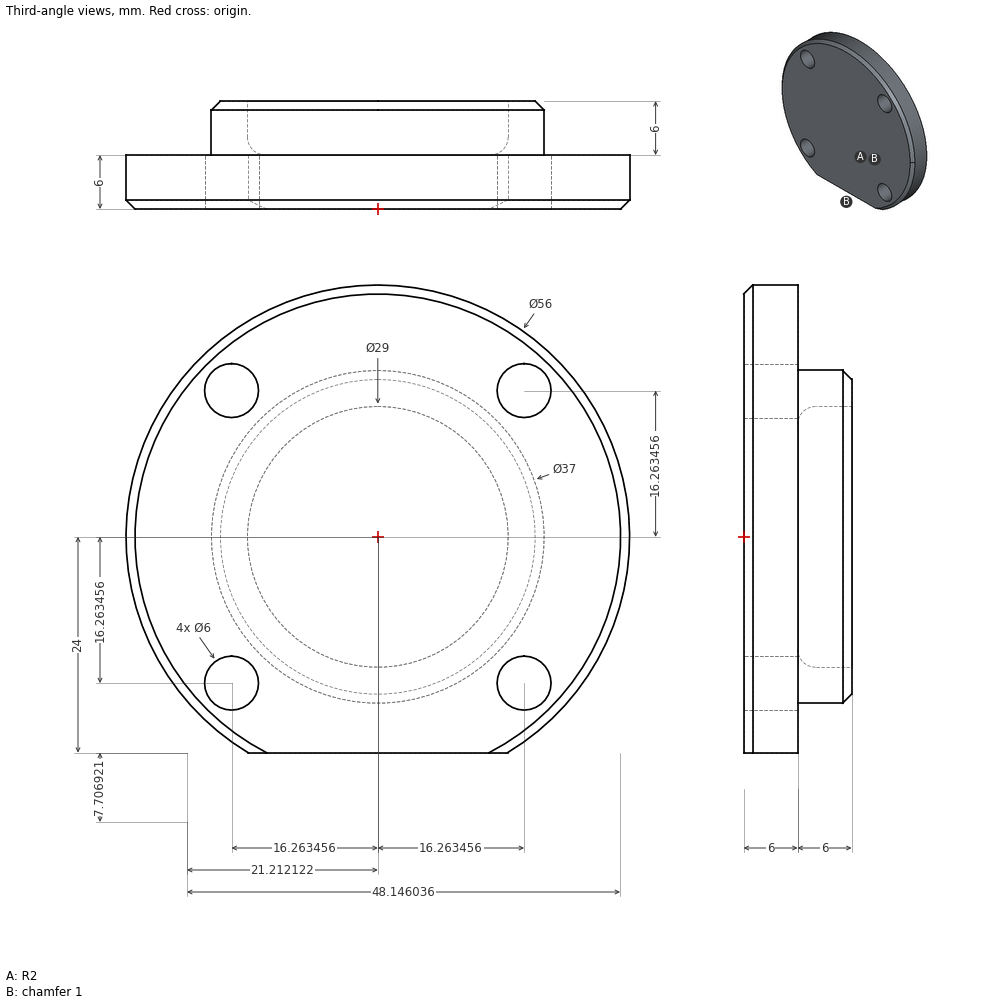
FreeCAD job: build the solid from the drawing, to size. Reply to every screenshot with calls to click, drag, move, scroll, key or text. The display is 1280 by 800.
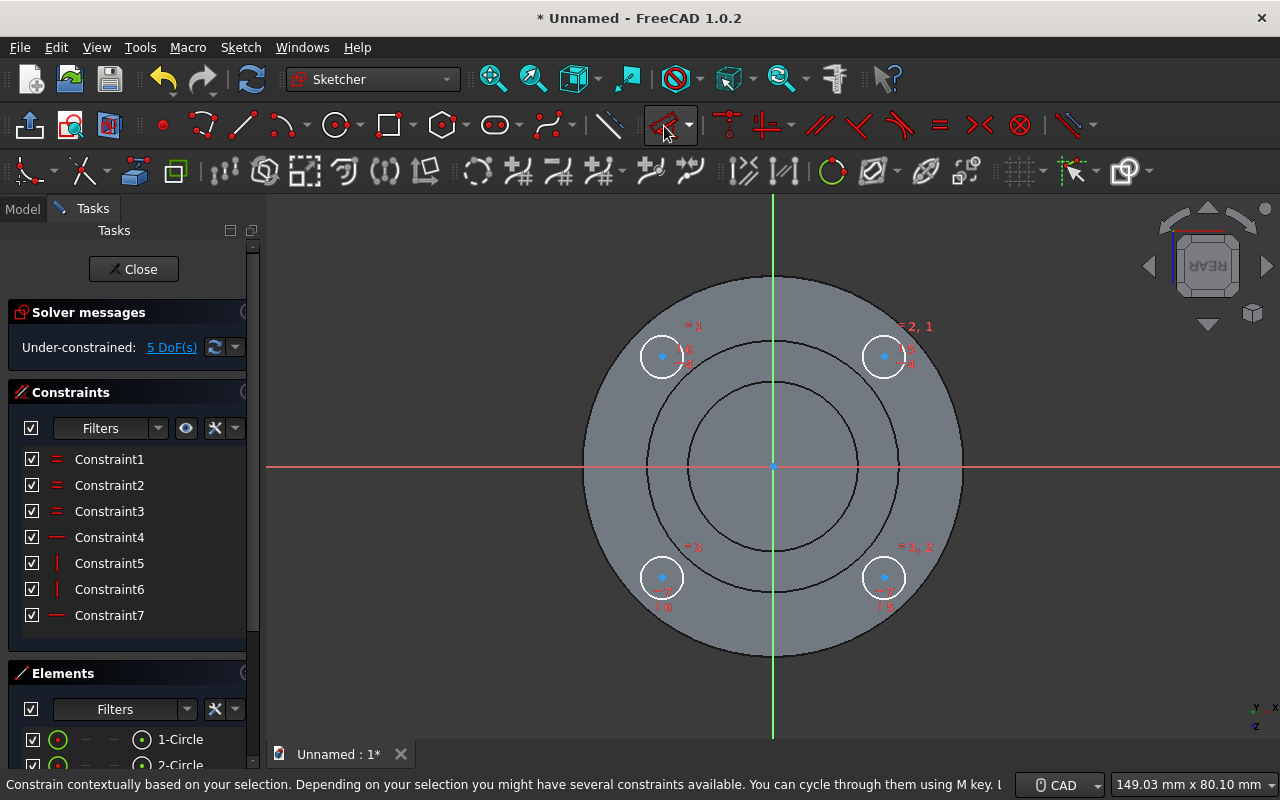
click(677, 342)
click(700, 319)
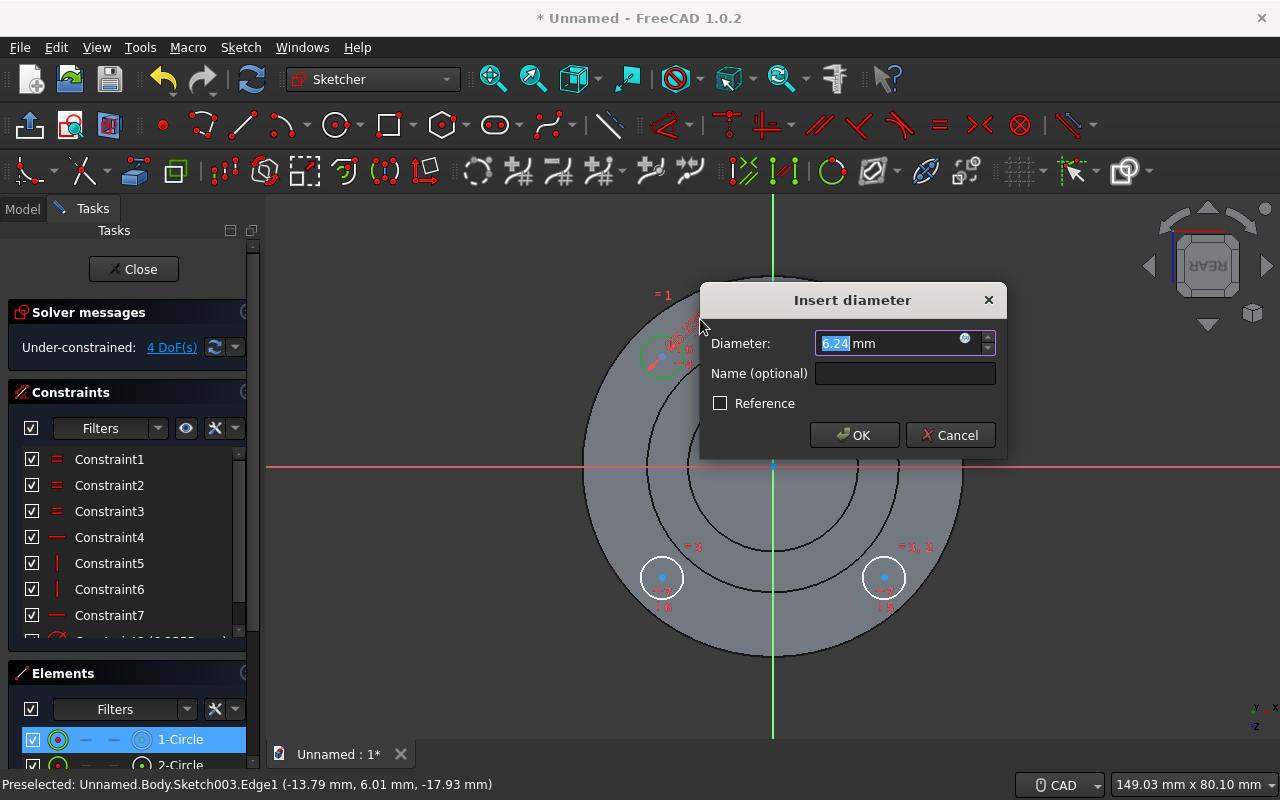
text(6)
key(Return)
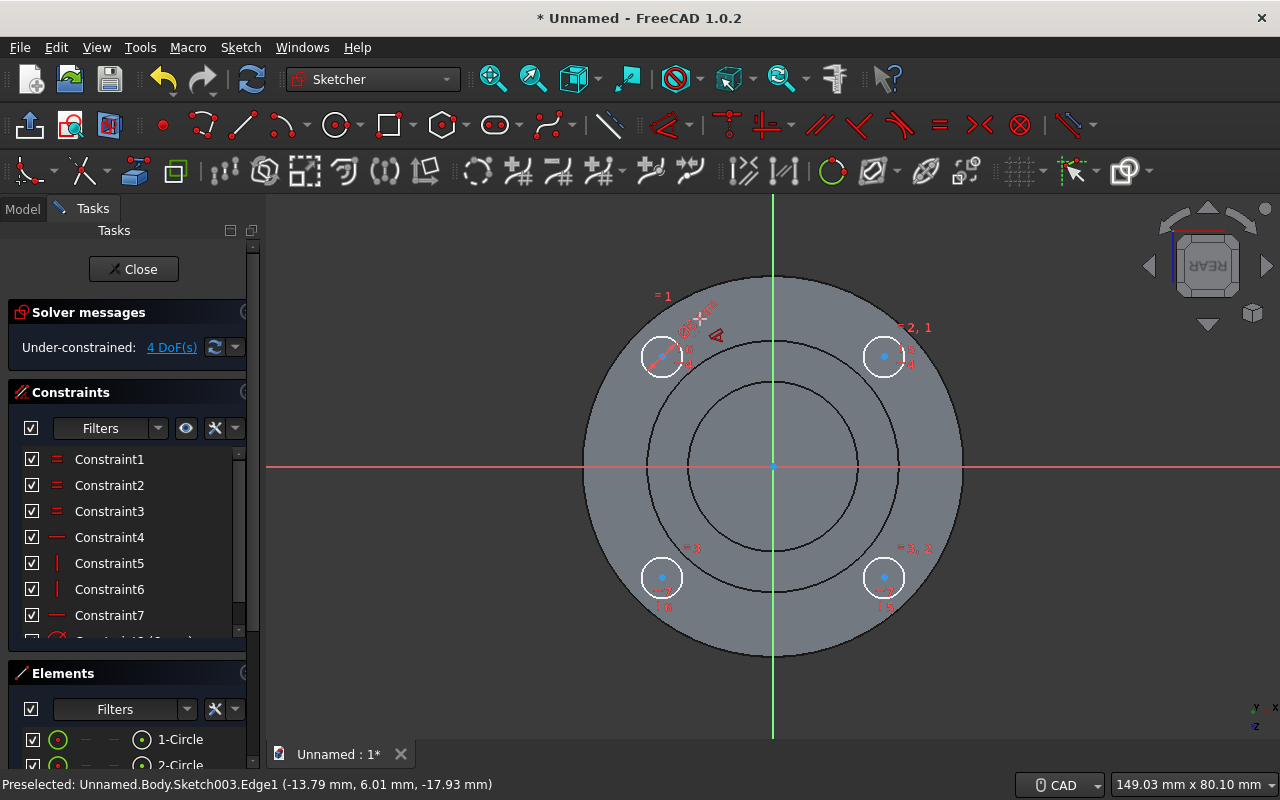
click(662, 357)
click(718, 501)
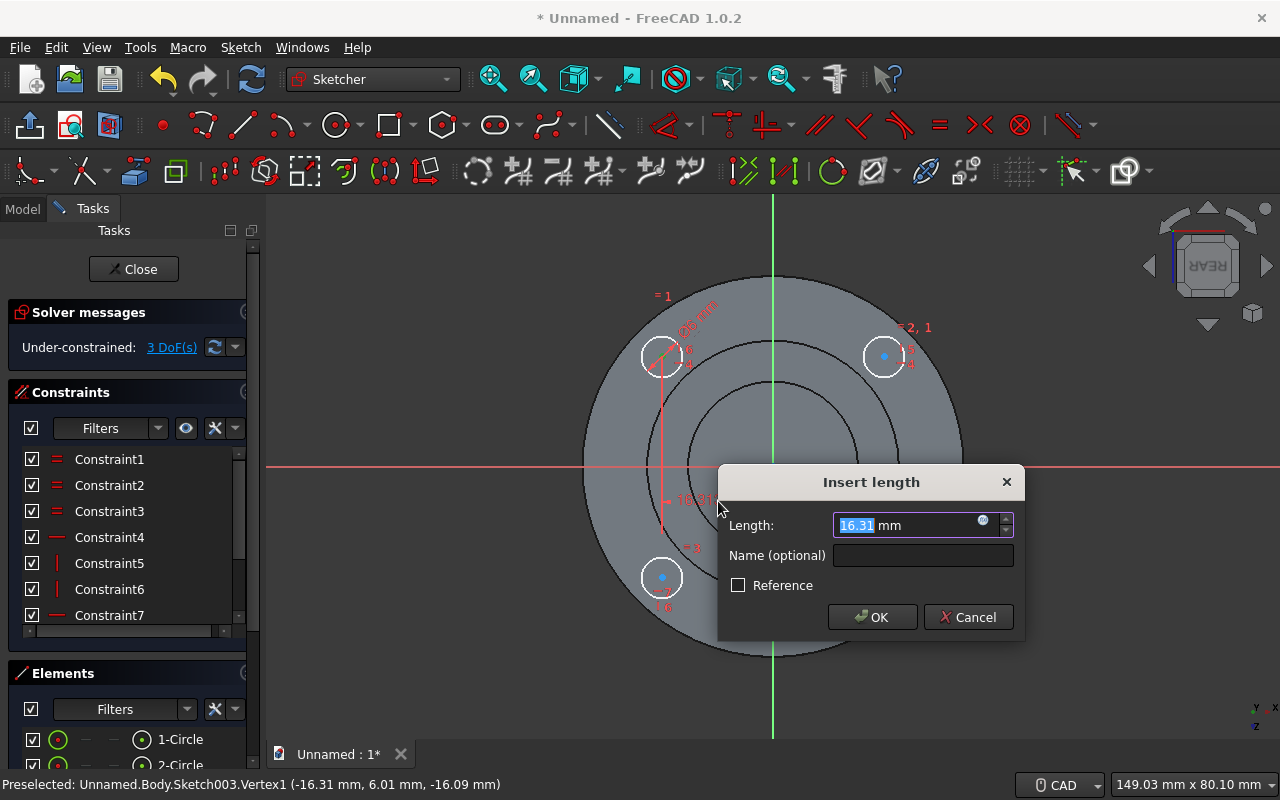
text(16.263456)
key(Return)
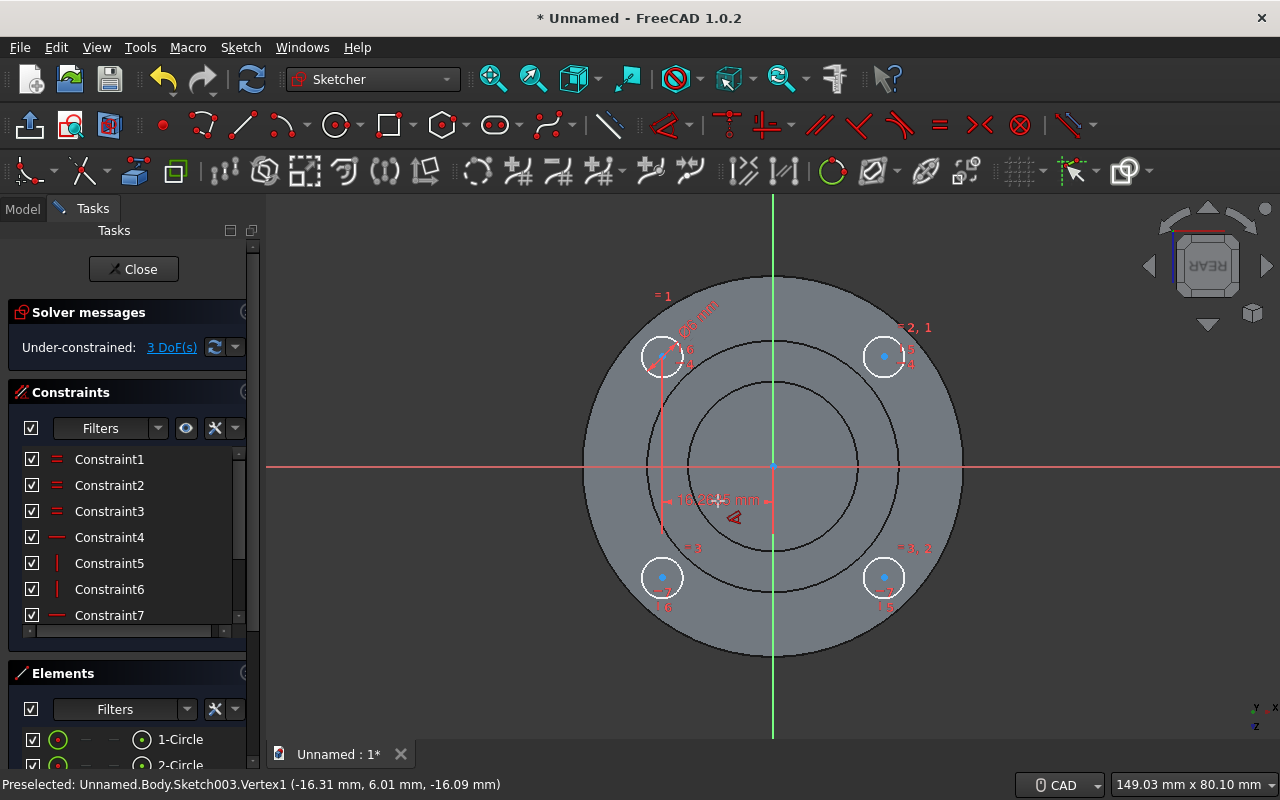
click(662, 357)
click(628, 412)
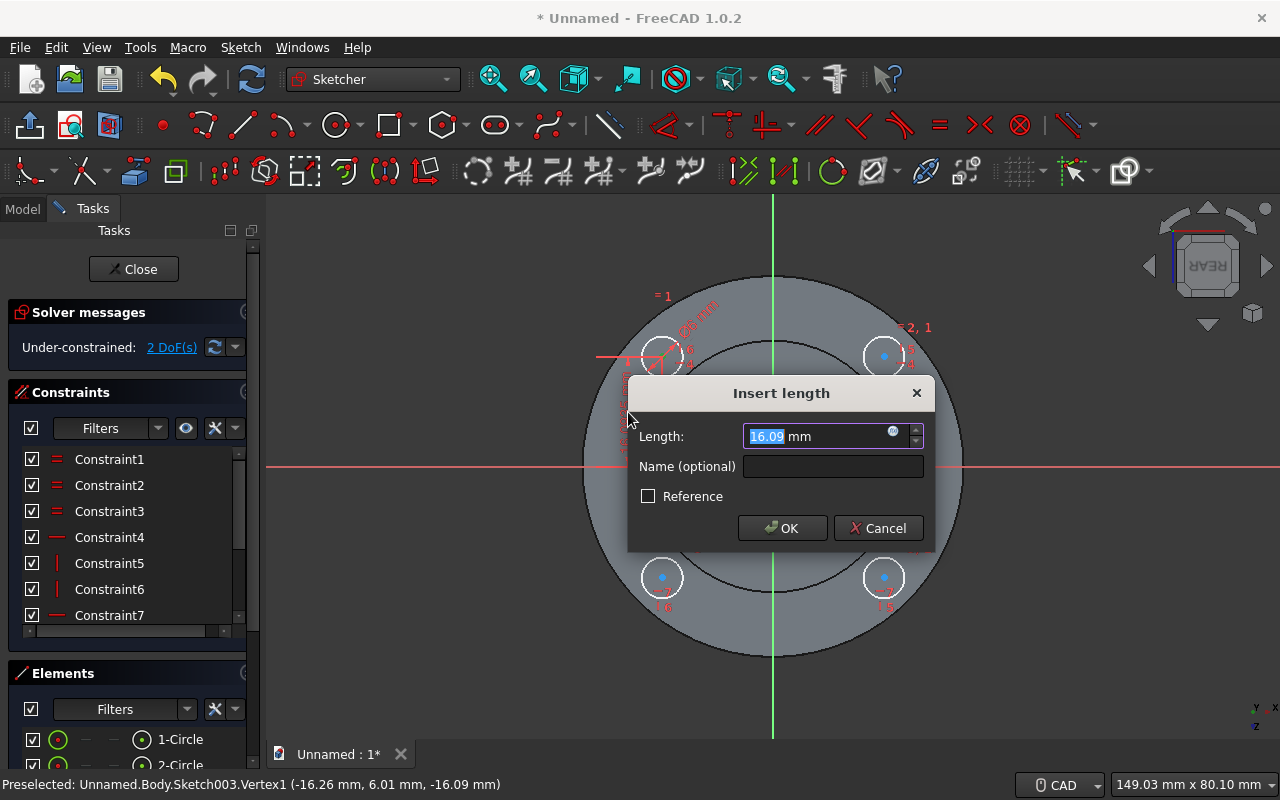
text(16.263456)
key(Return)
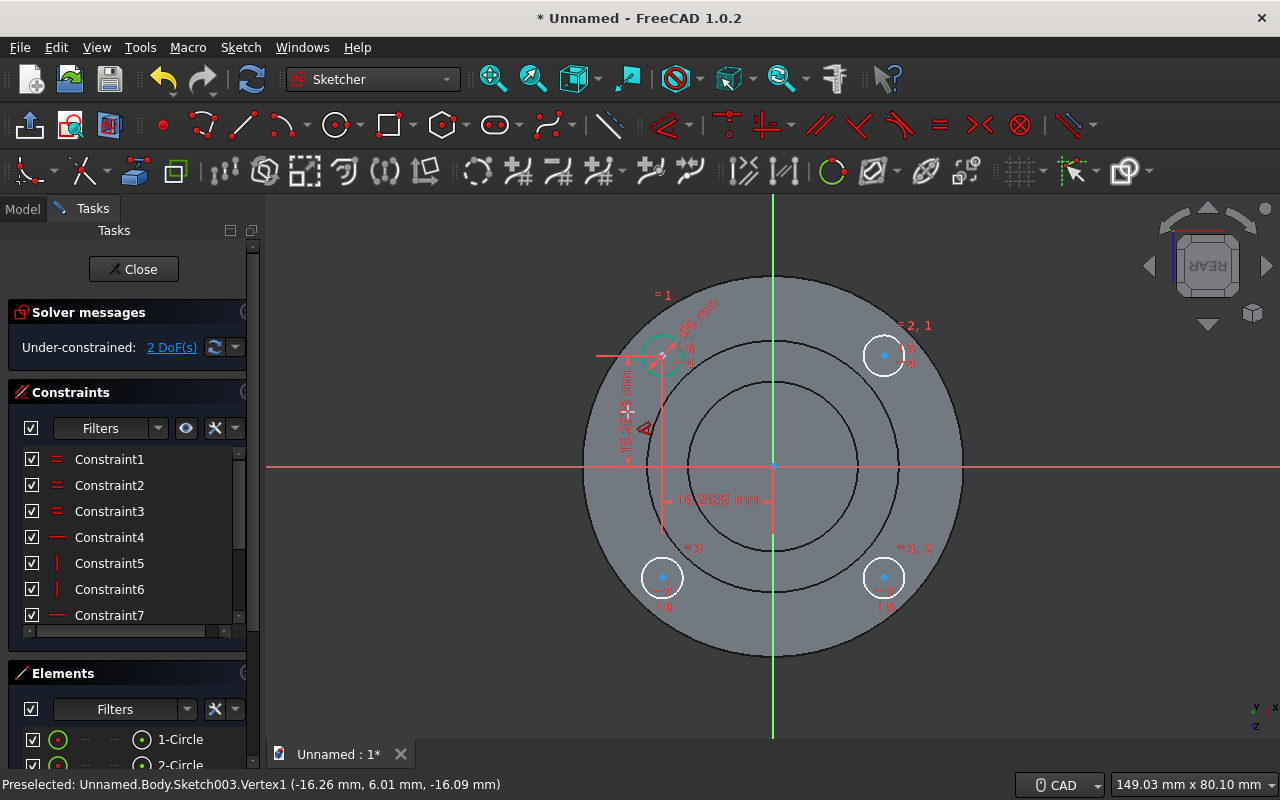
click(884, 356)
click(828, 322)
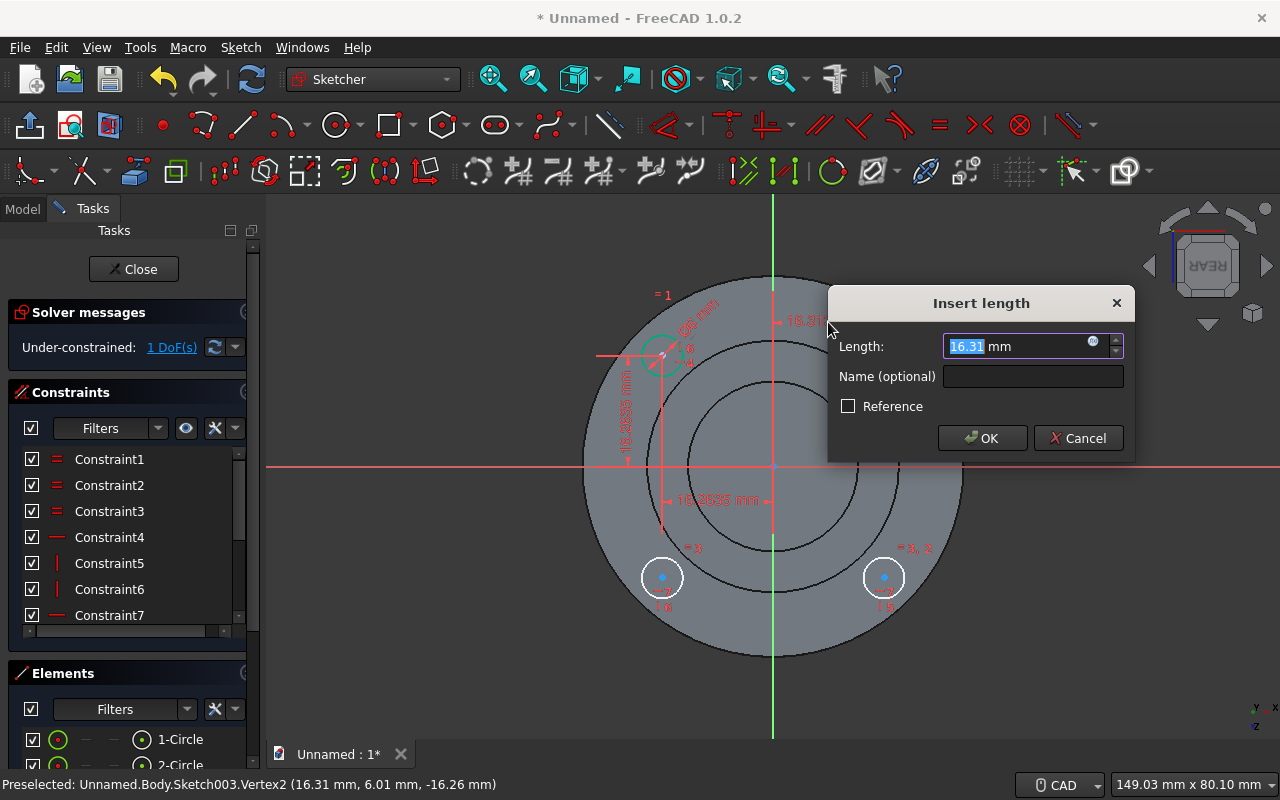
text(16.263456)
key(Return)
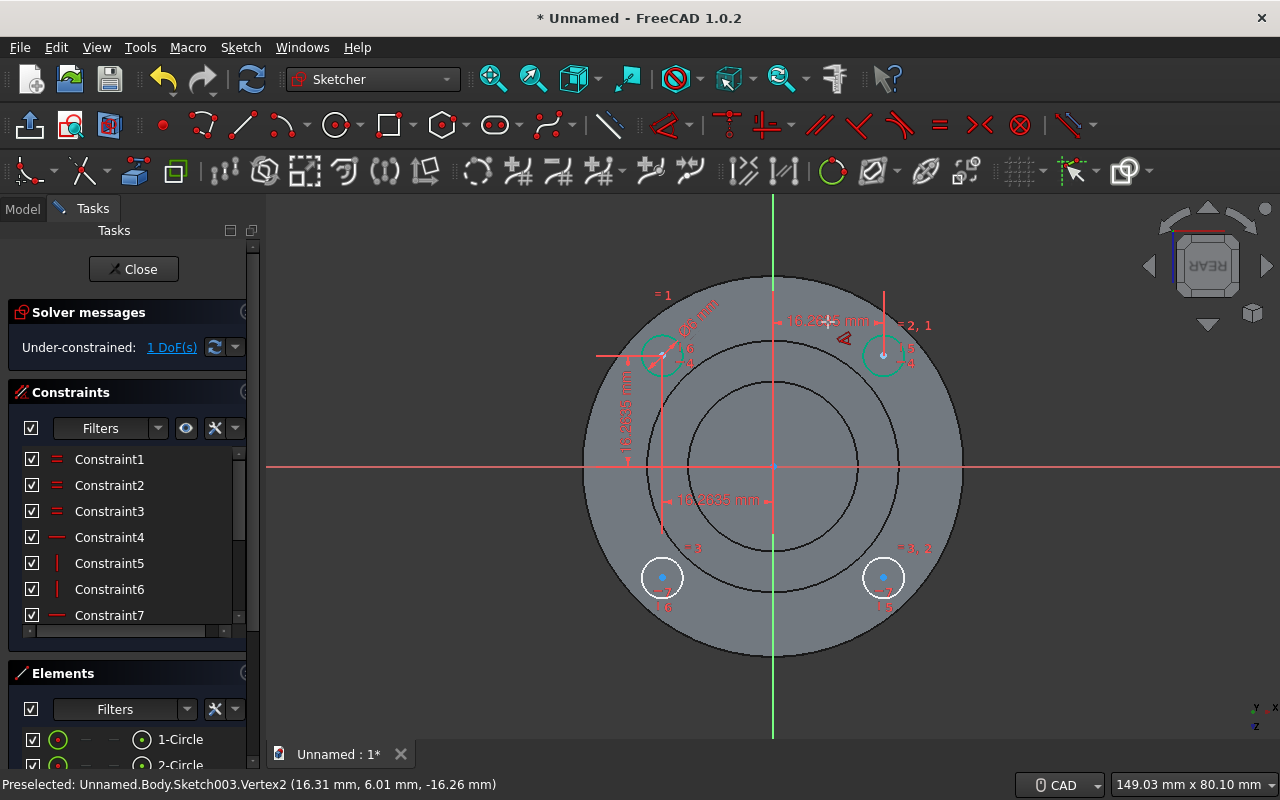
click(884, 578)
click(918, 522)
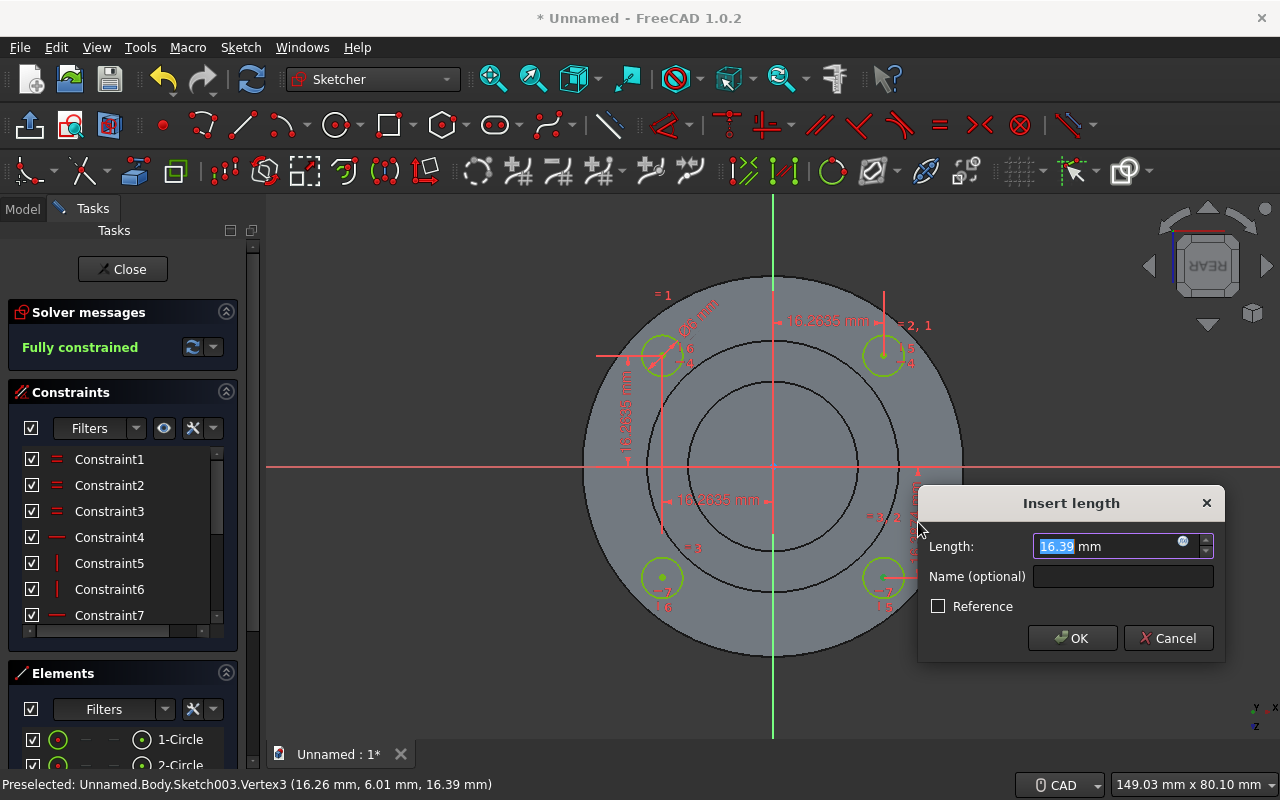
text(16.263456)
key(Return)
key(Escape)